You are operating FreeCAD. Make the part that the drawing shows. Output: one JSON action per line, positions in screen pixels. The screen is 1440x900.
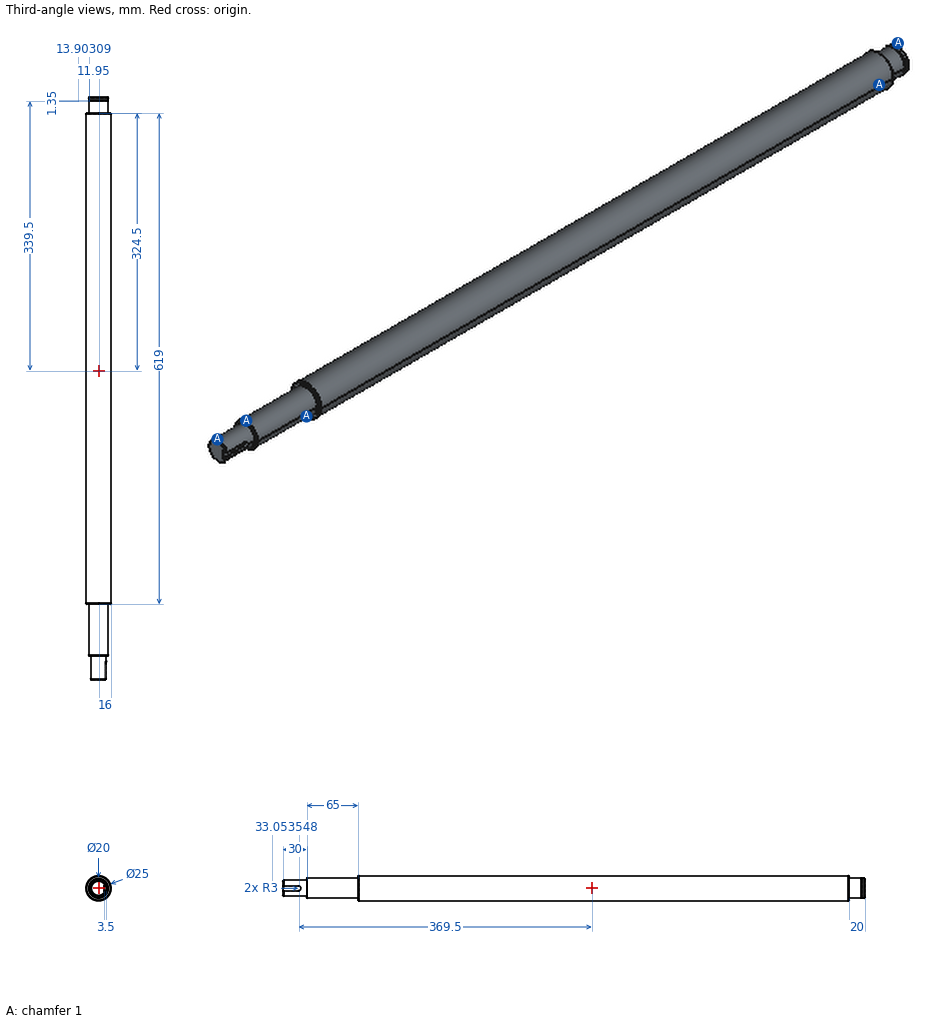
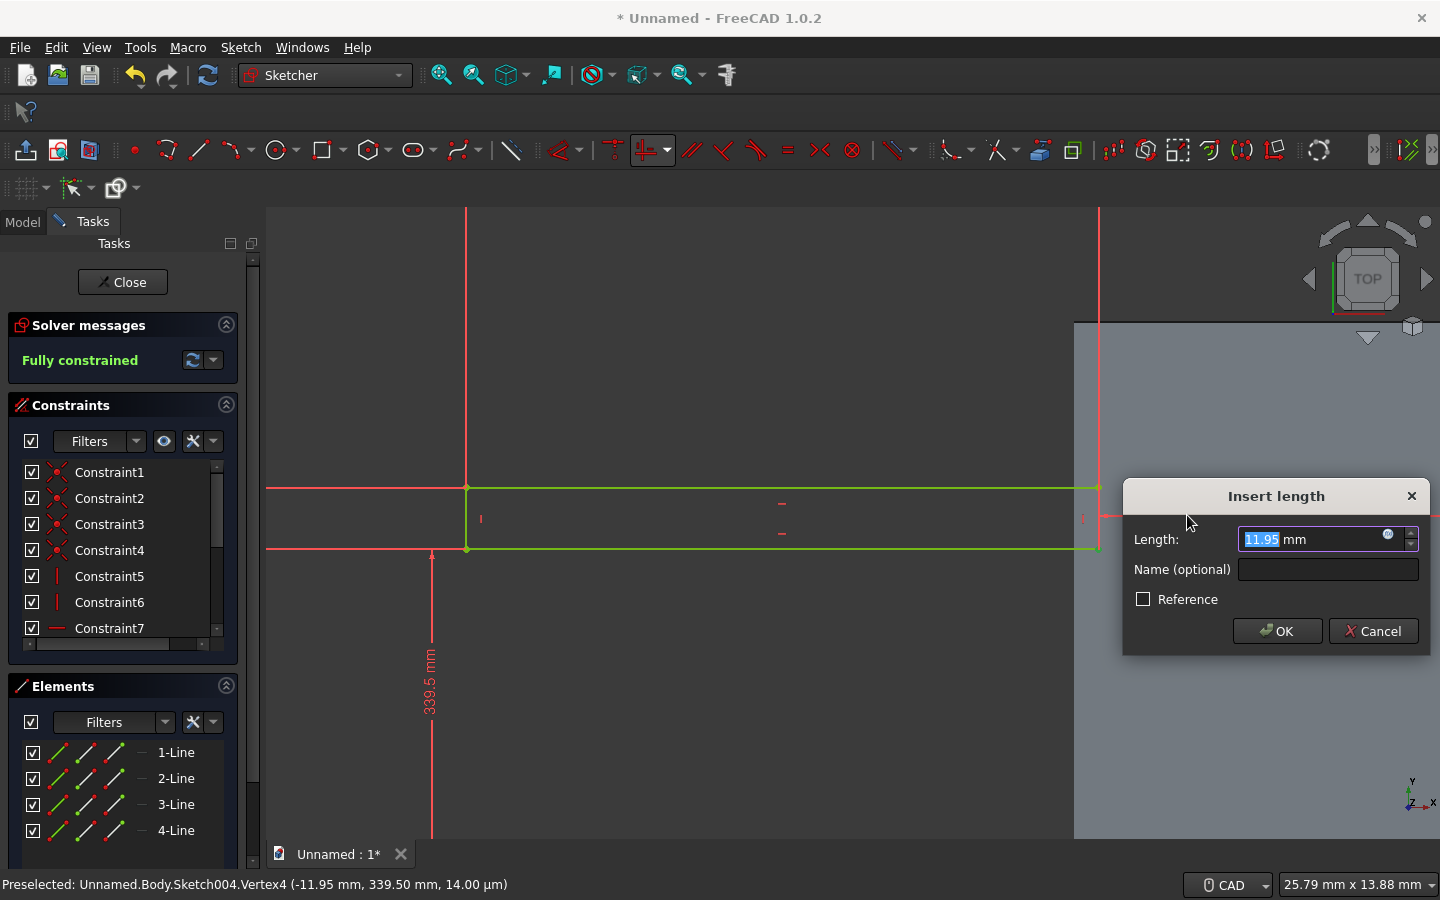
{"action": "type", "text": "11.95"}
{"action": "key", "text": "Return"}
{"action": "key", "text": "Escape"}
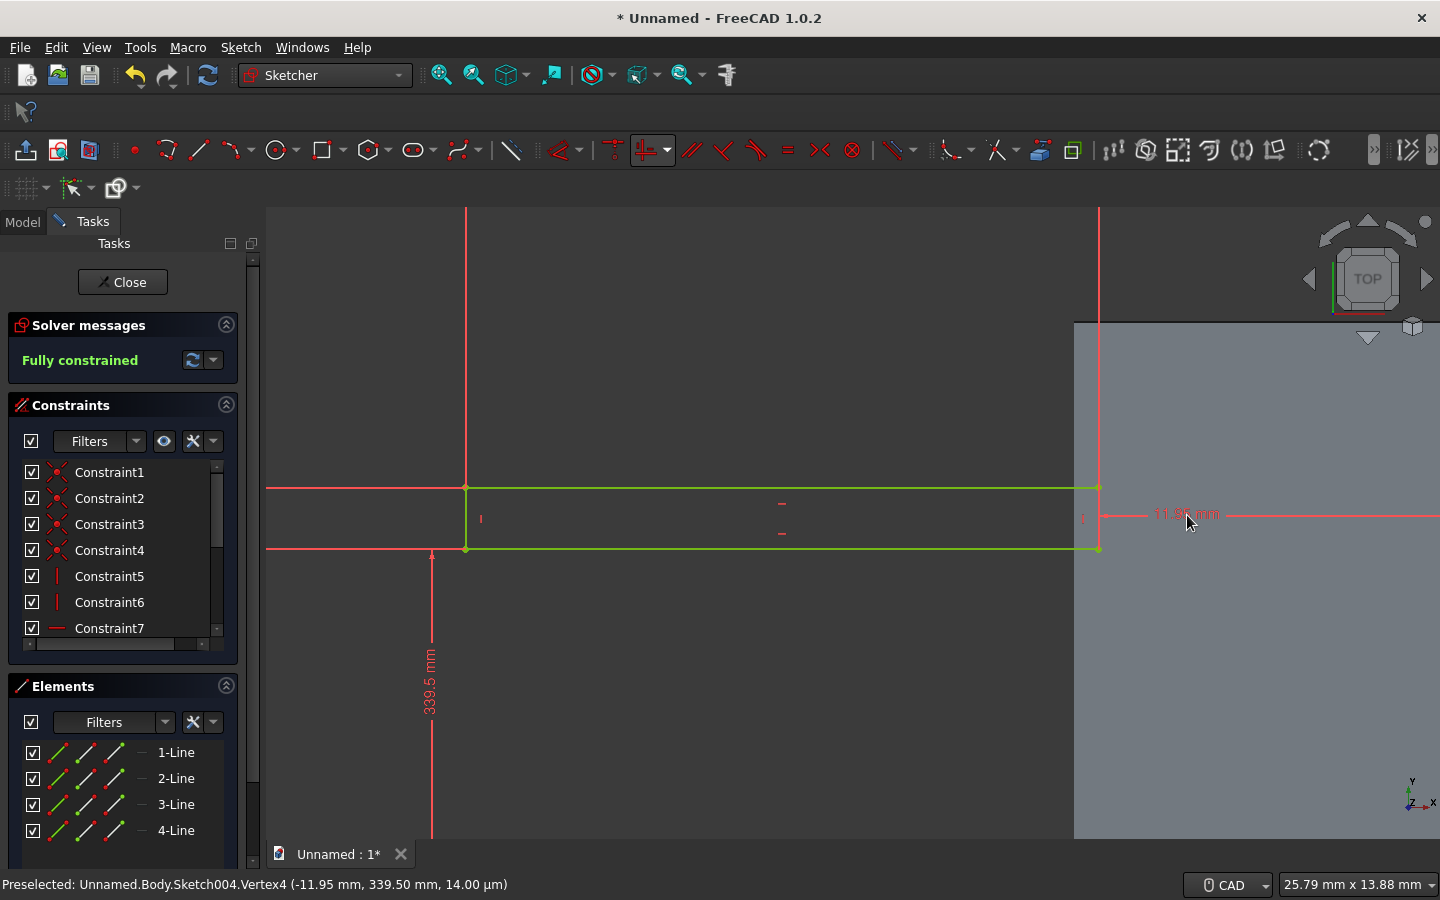
{"action": "left_click", "coordinate": [123, 282]}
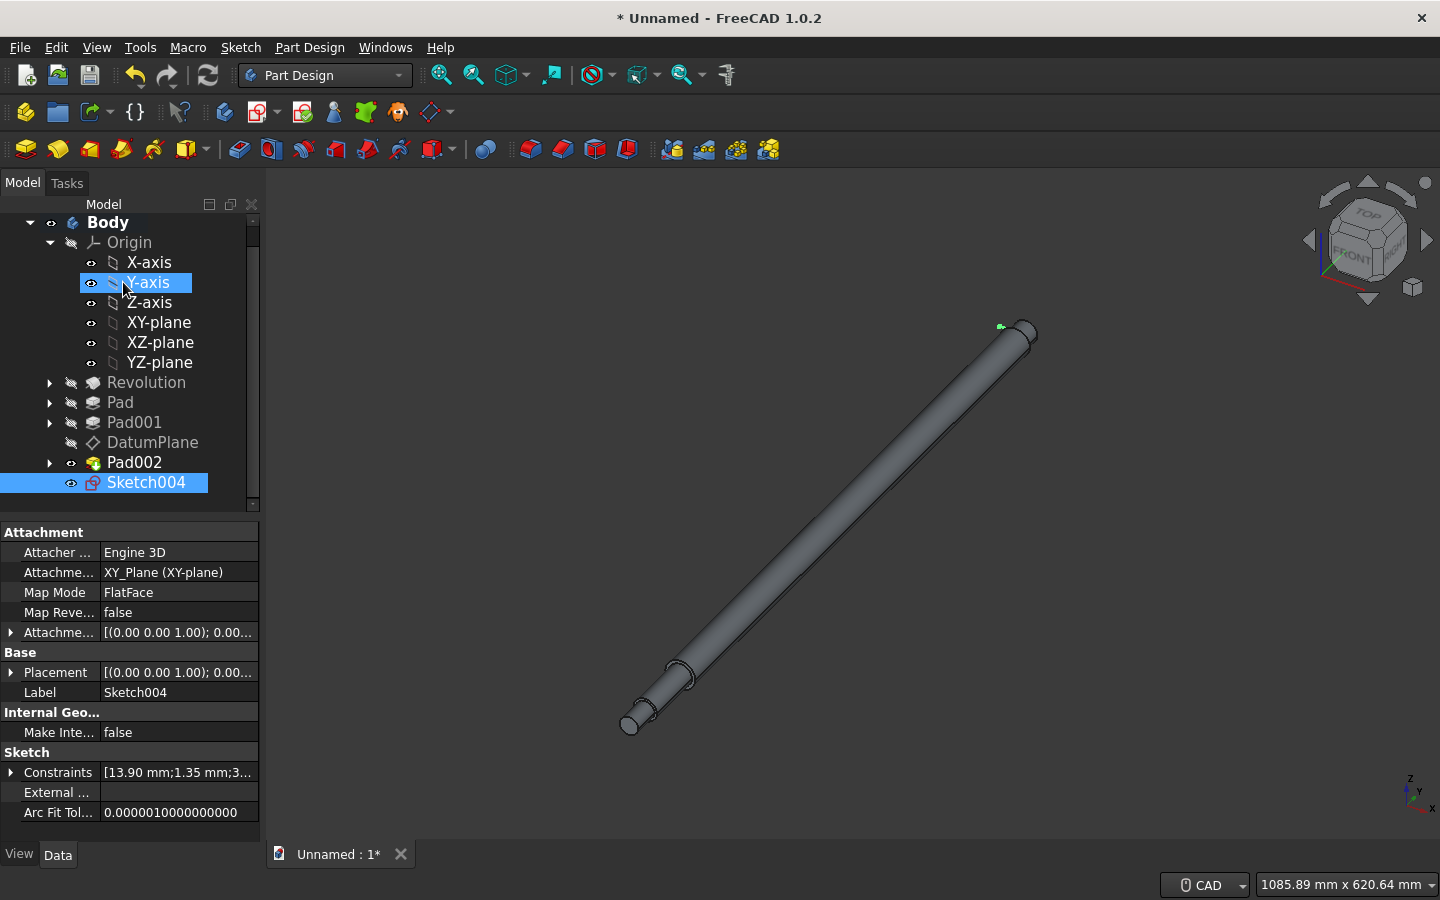
{"action": "left_click", "coordinate": [304, 150]}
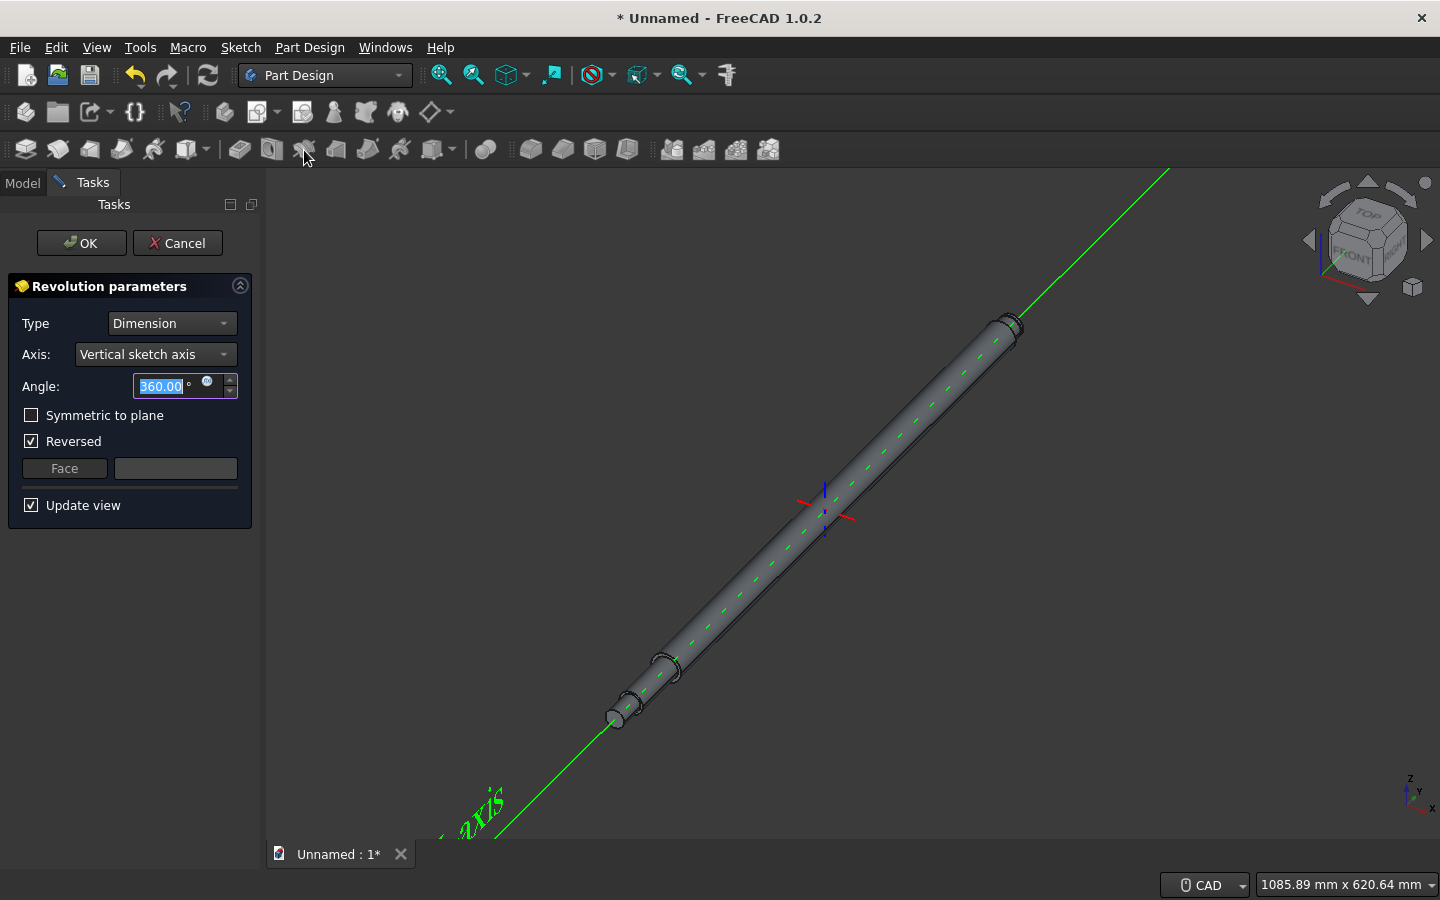
{"action": "left_click", "coordinate": [82, 243]}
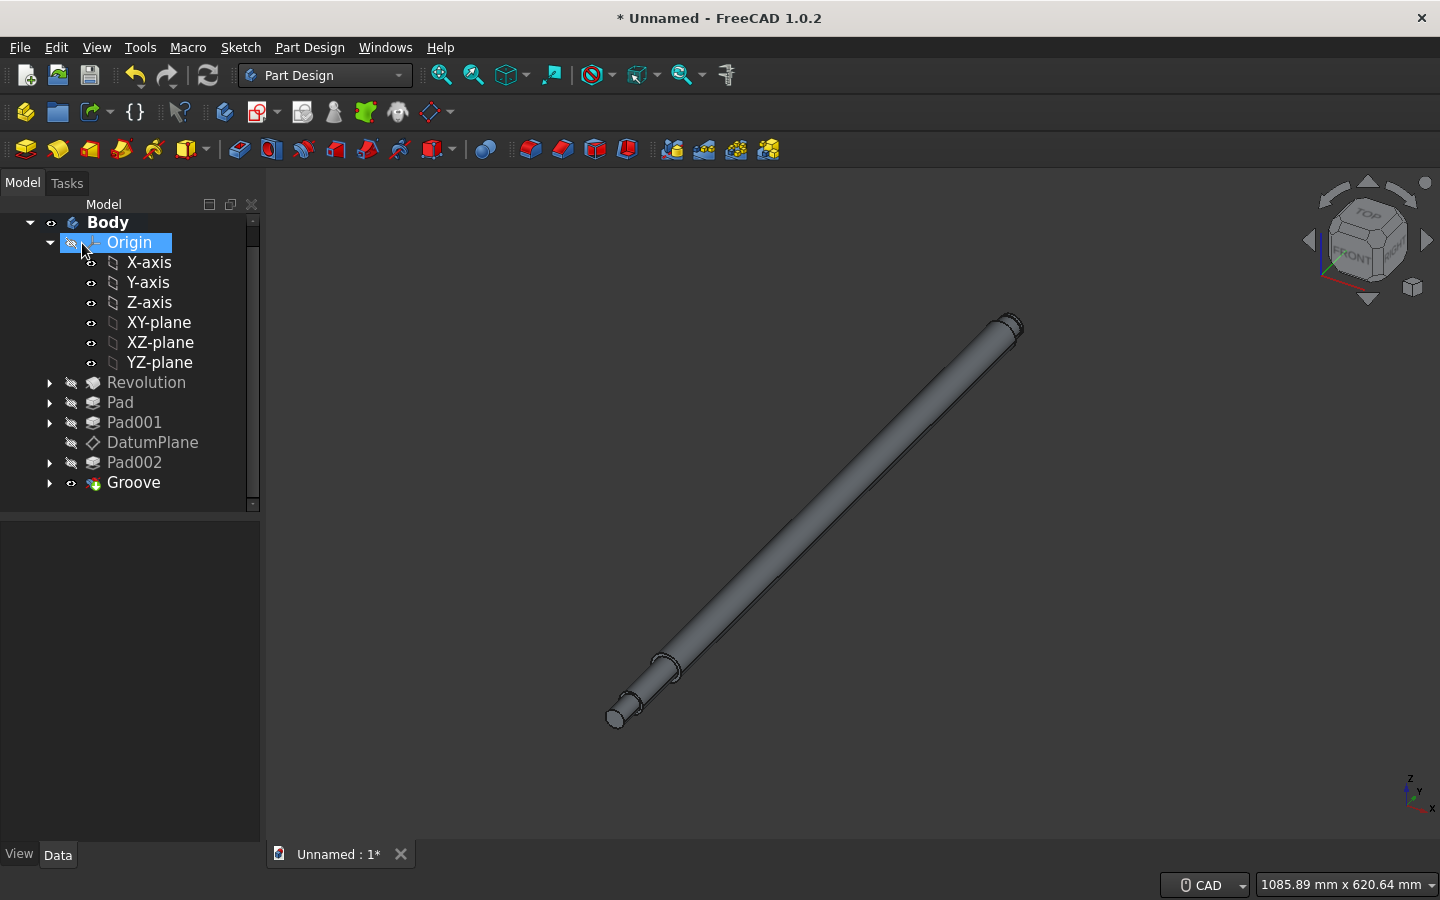
{"action": "left_click", "coordinate": [622, 693]}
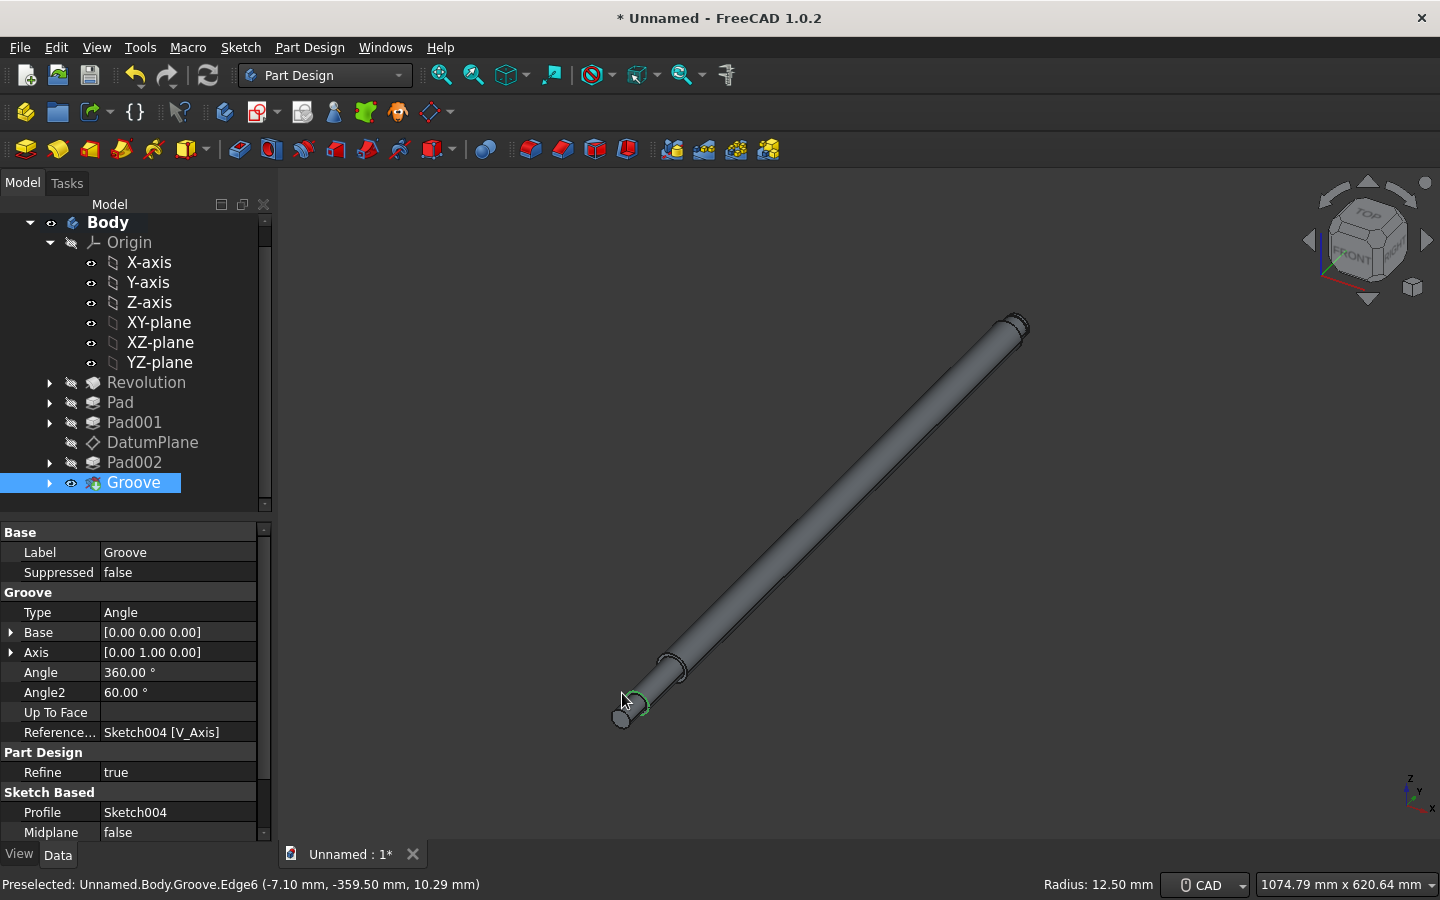
{"action": "left_click", "coordinate": [611, 715], "text": "ctrl"}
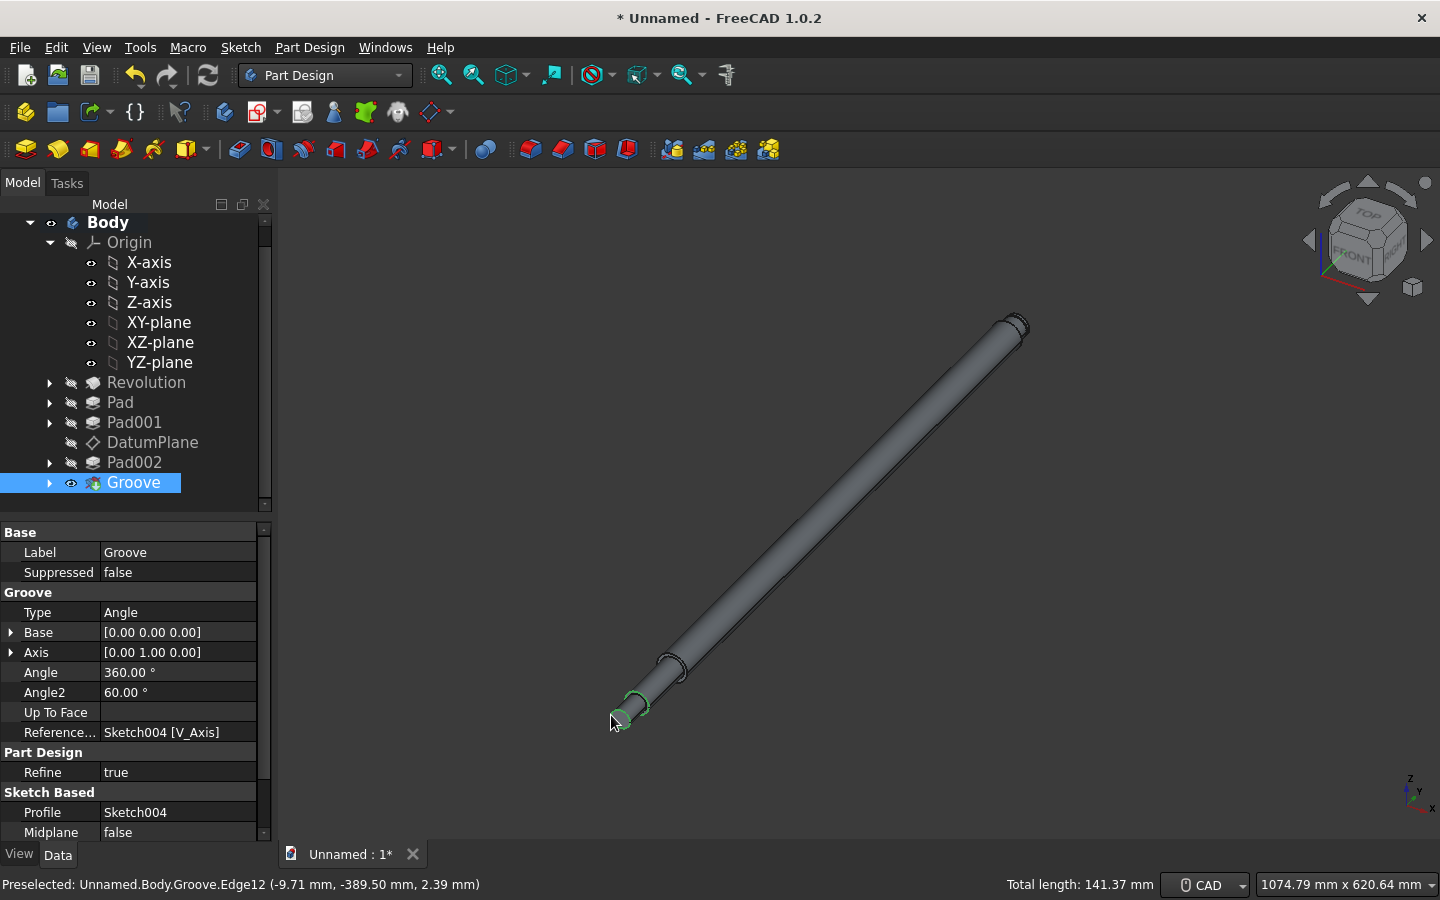
{"action": "left_click", "coordinate": [1022, 337], "text": "ctrl"}